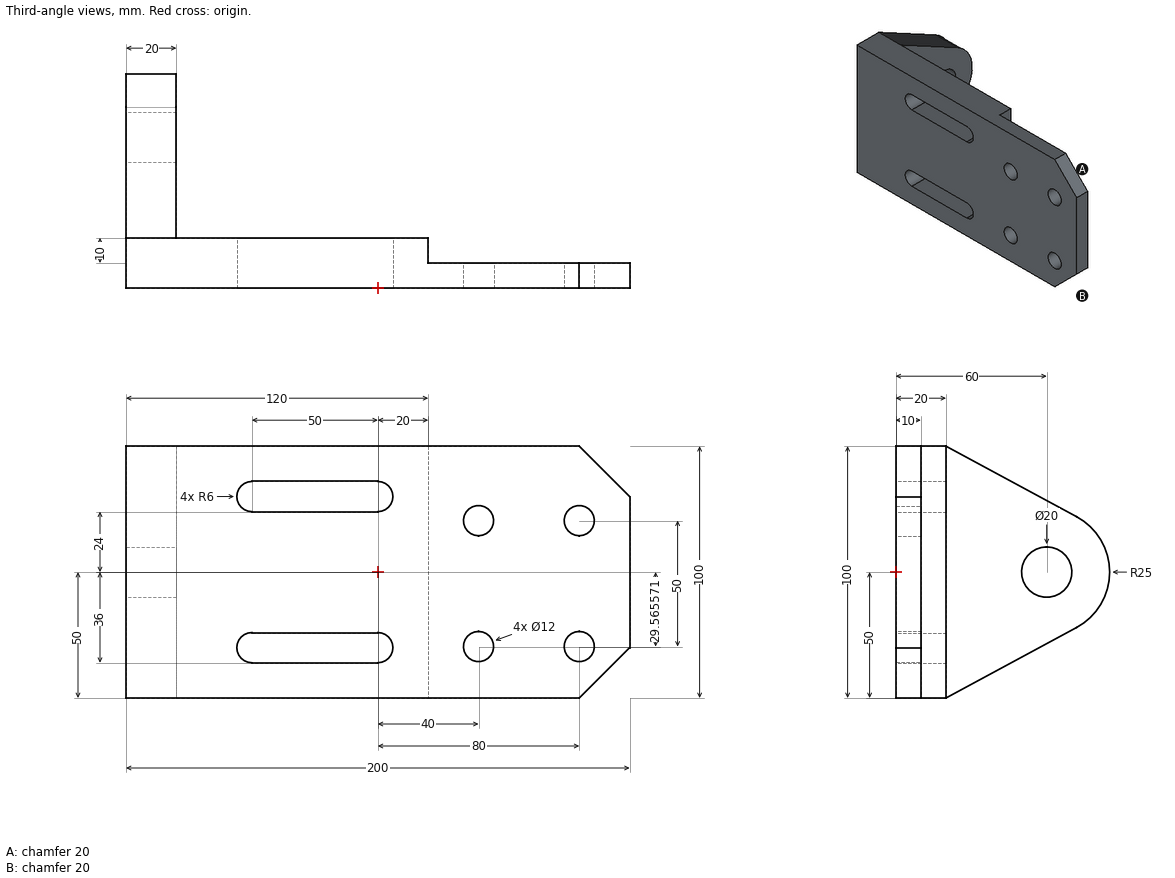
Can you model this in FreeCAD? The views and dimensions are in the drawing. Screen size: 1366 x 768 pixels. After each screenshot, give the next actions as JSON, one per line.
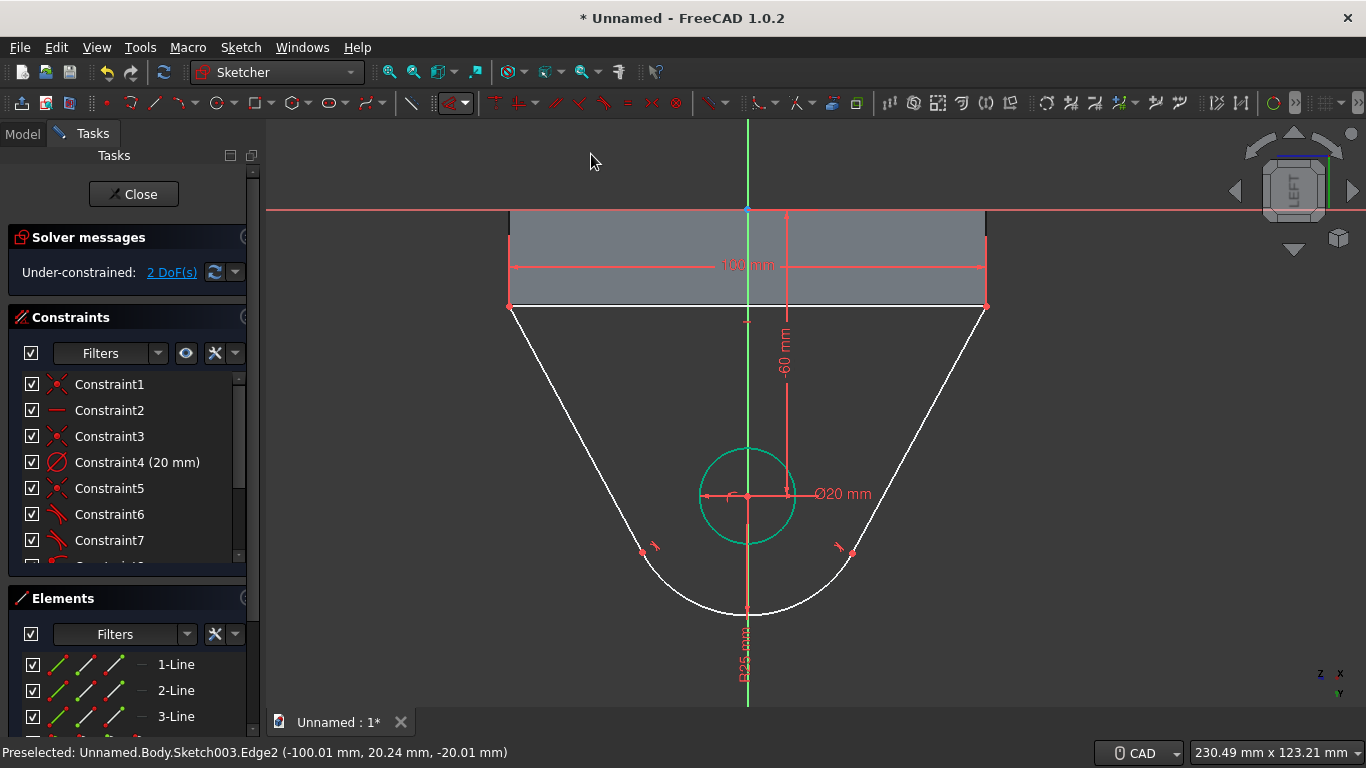
{"action": "left_click", "coordinate": [986, 306]}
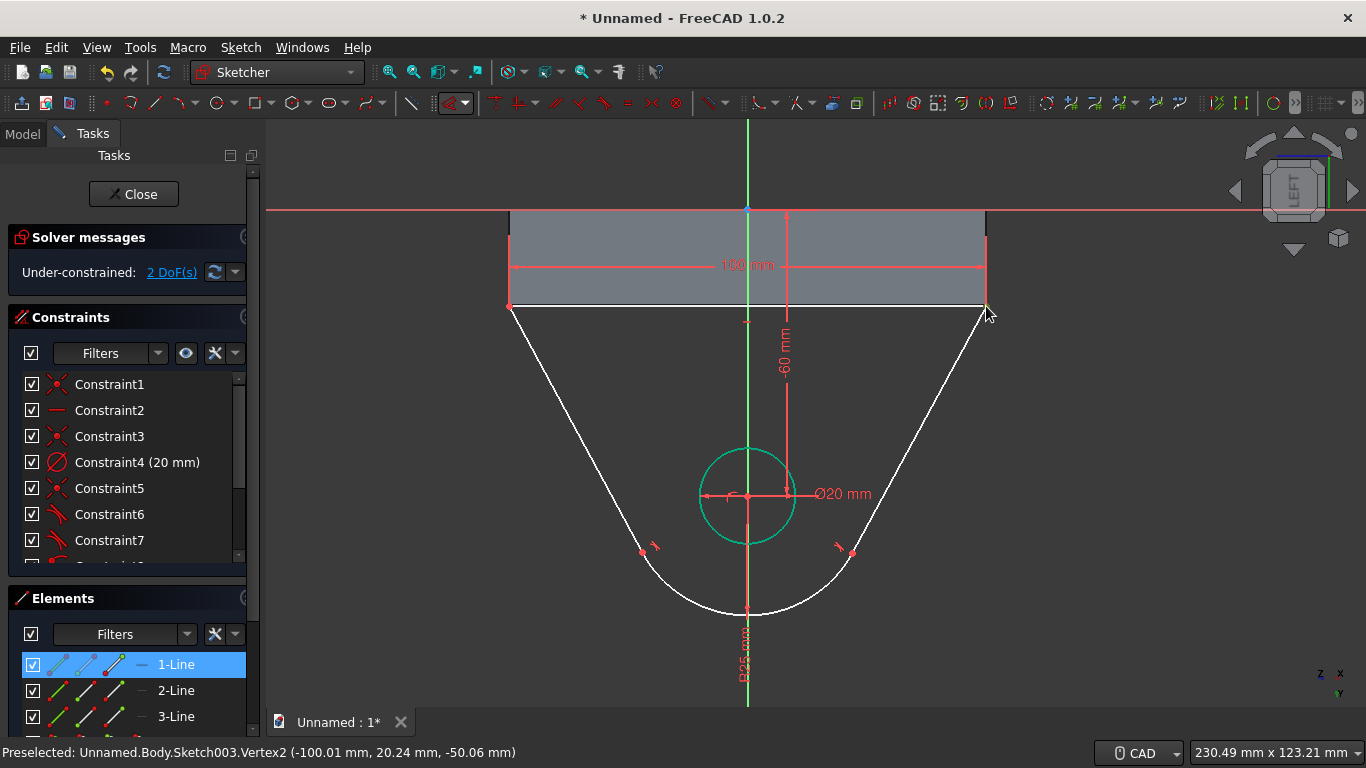
{"action": "key", "text": "l"}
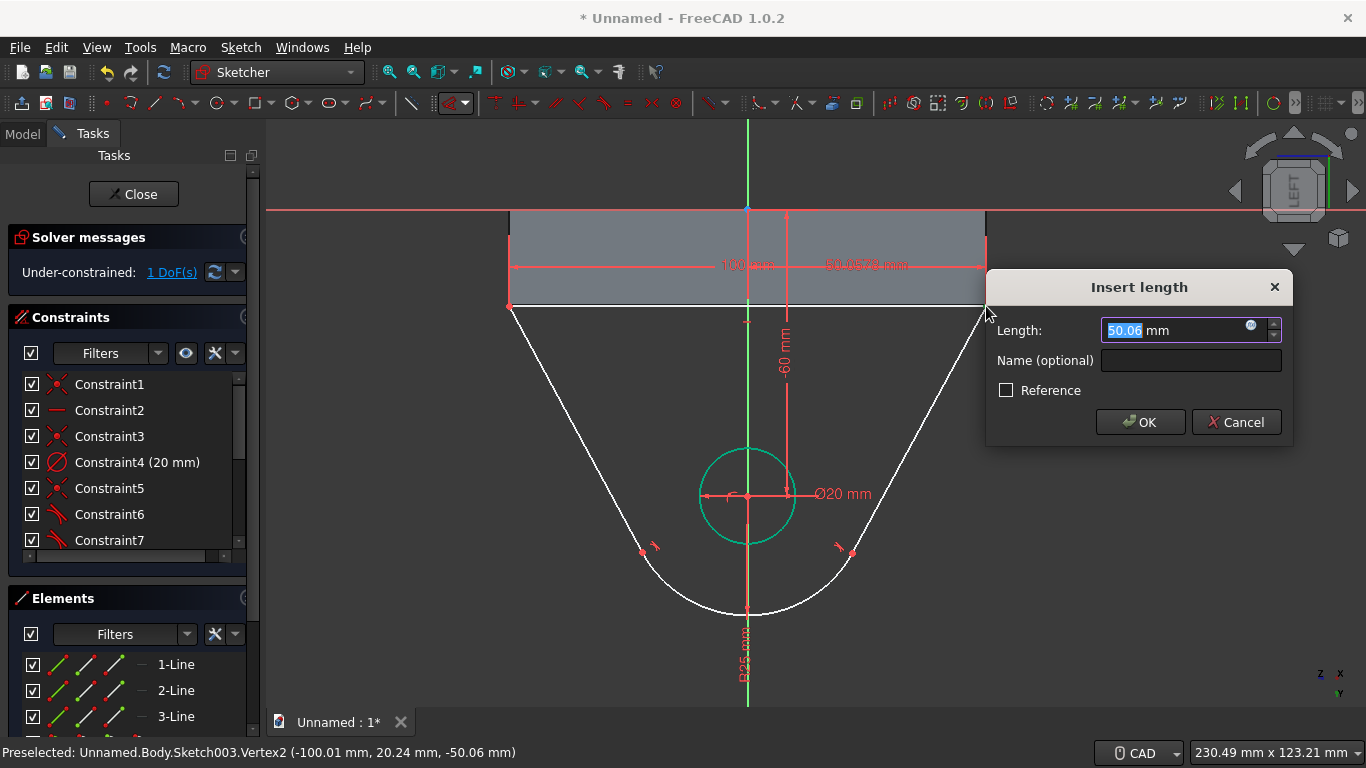
{"action": "type", "text": "50"}
{"action": "key", "text": "Return"}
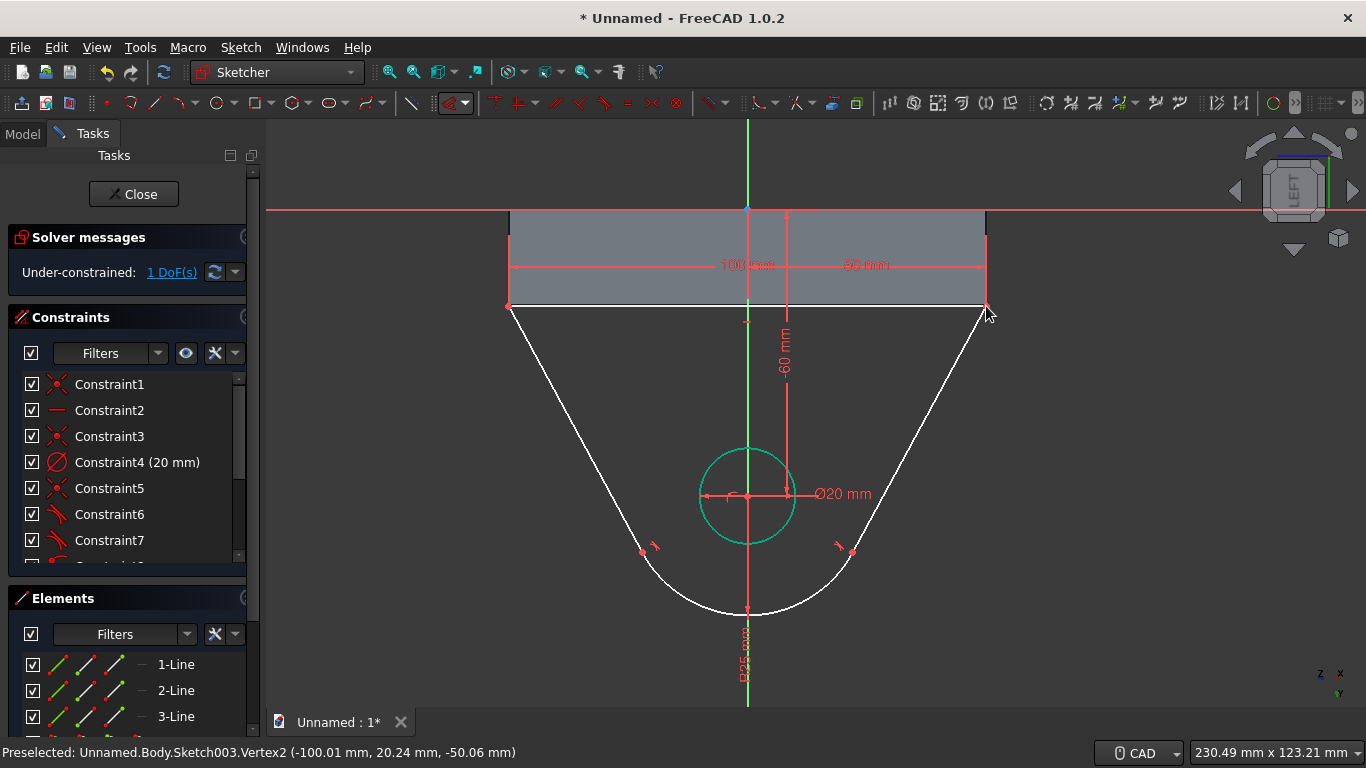
{"action": "left_click", "coordinate": [986, 306]}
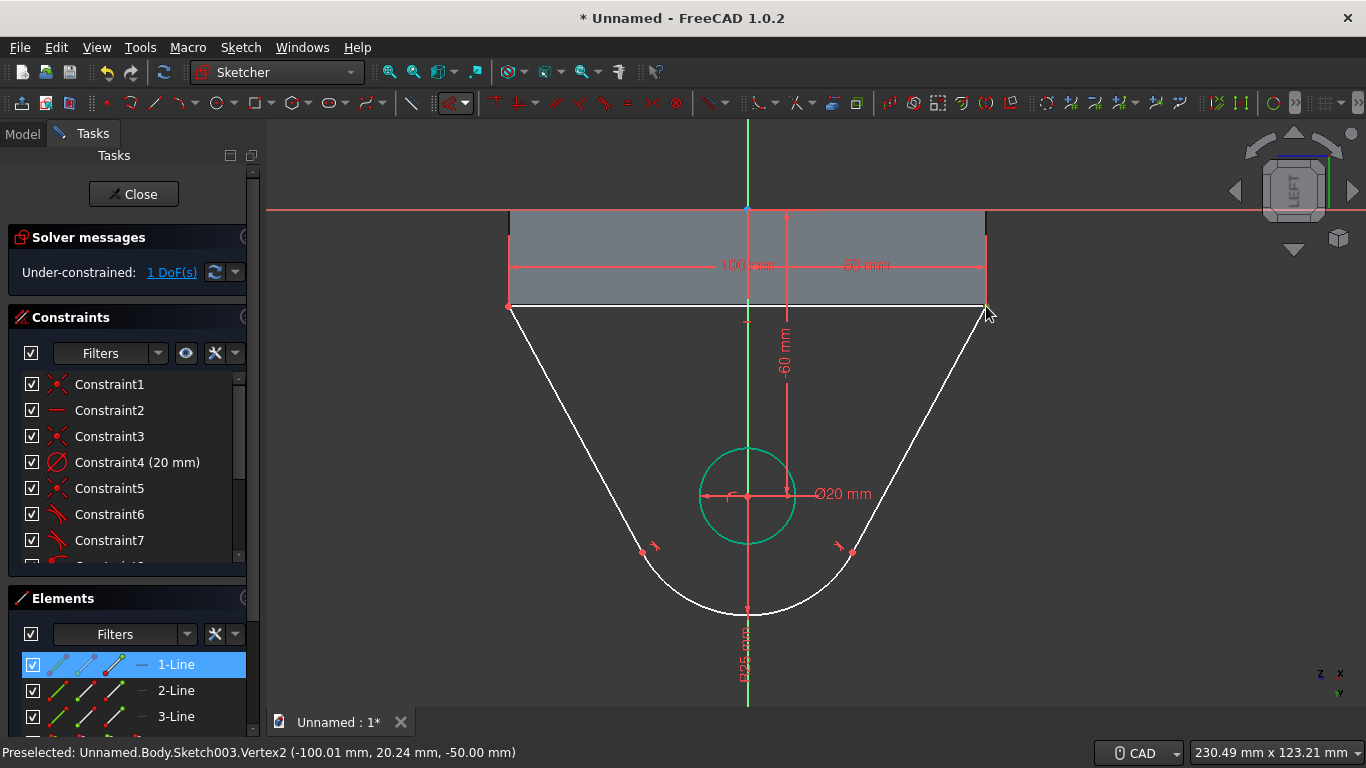
{"action": "left_click", "coordinate": [468, 104]}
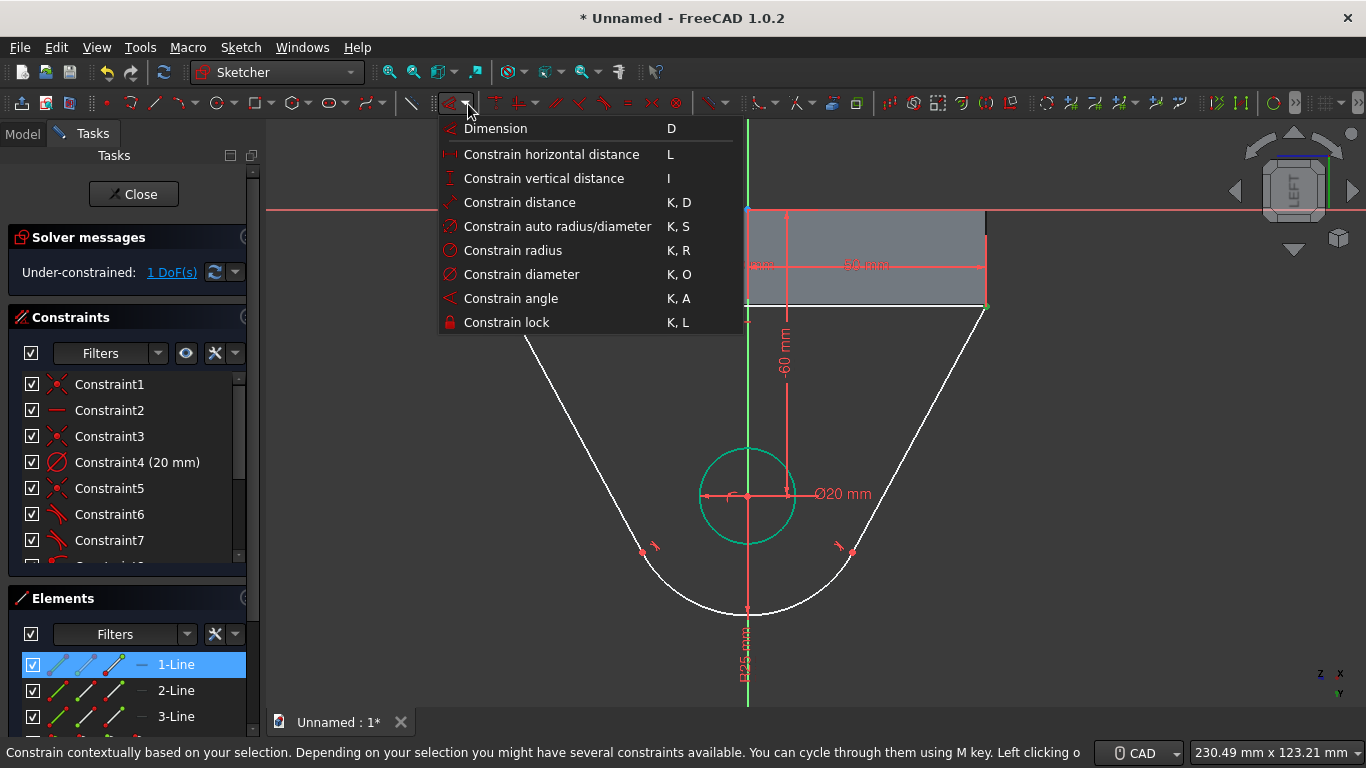
{"action": "left_click", "coordinate": [591, 178]}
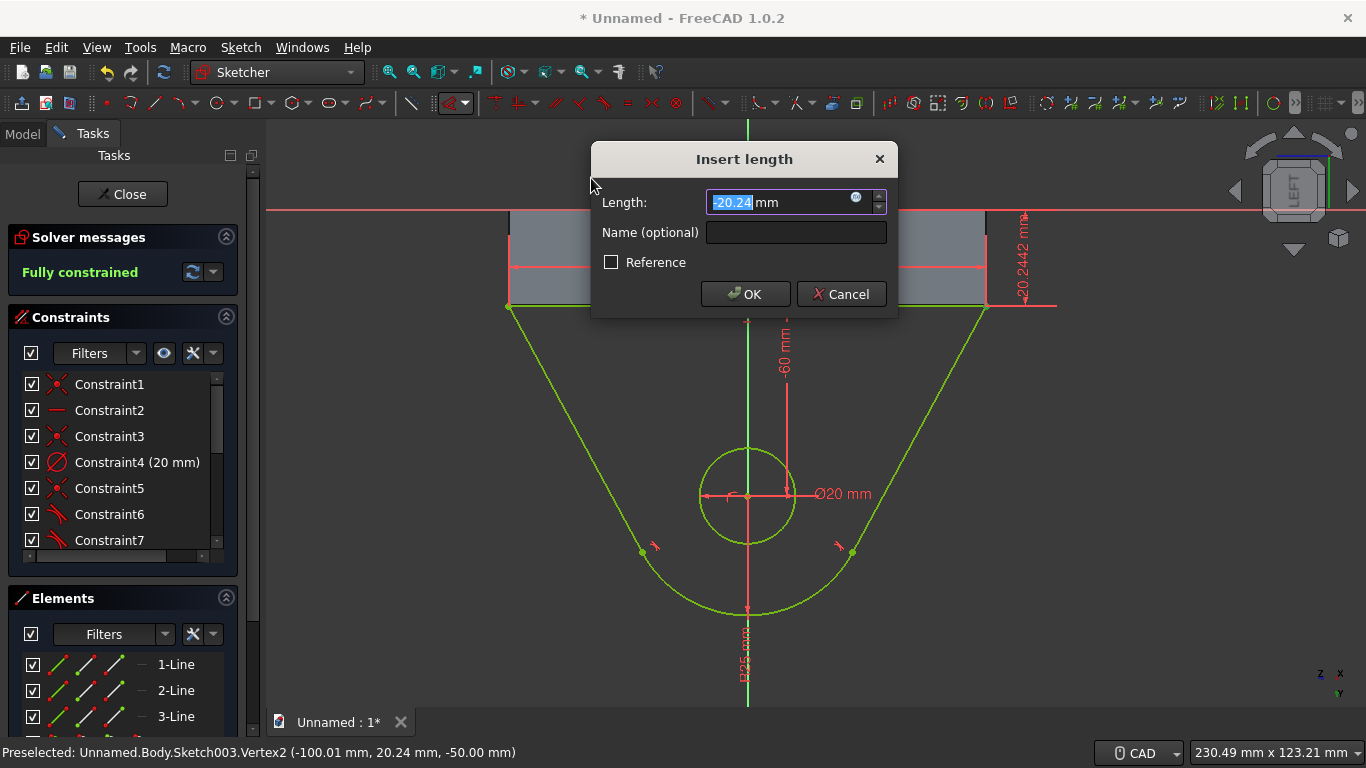
{"action": "type", "text": "-20"}
{"action": "key", "text": "Return"}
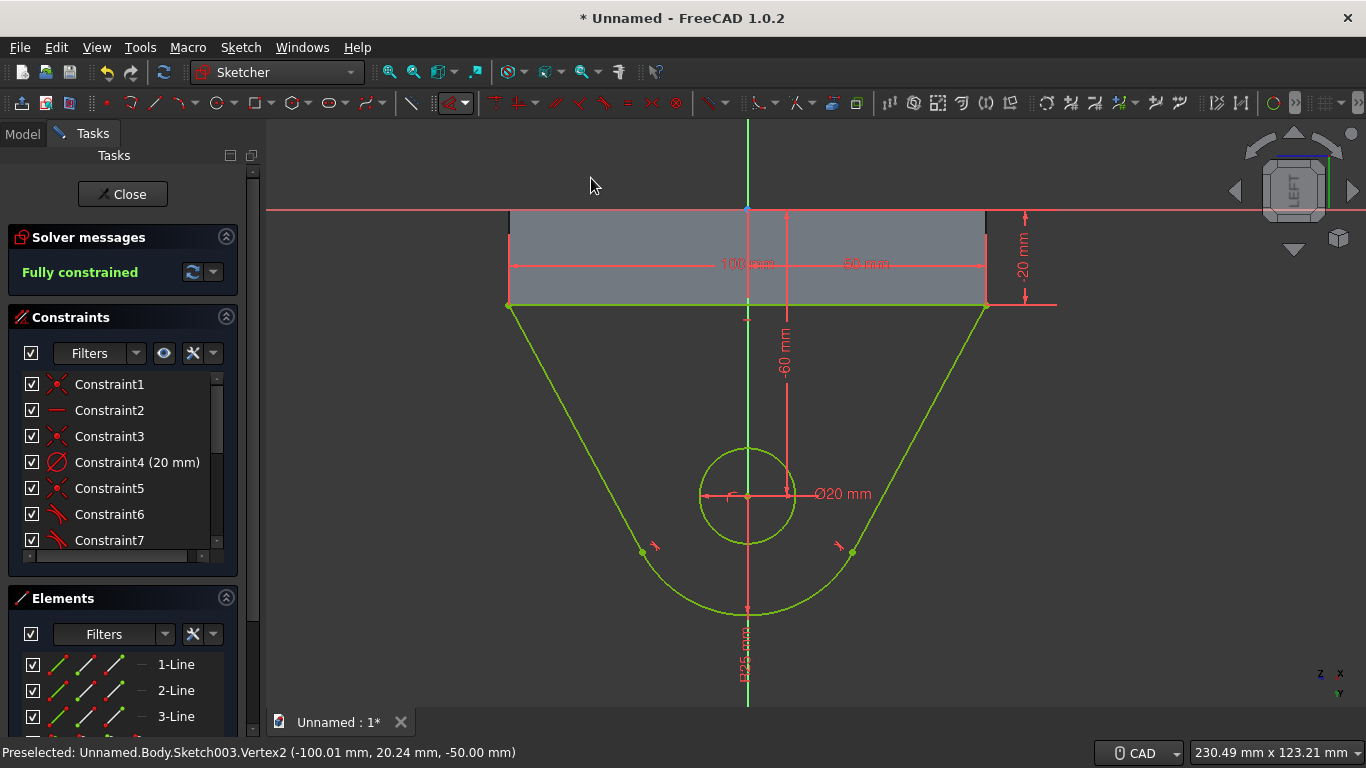
{"action": "left_click", "coordinate": [123, 194]}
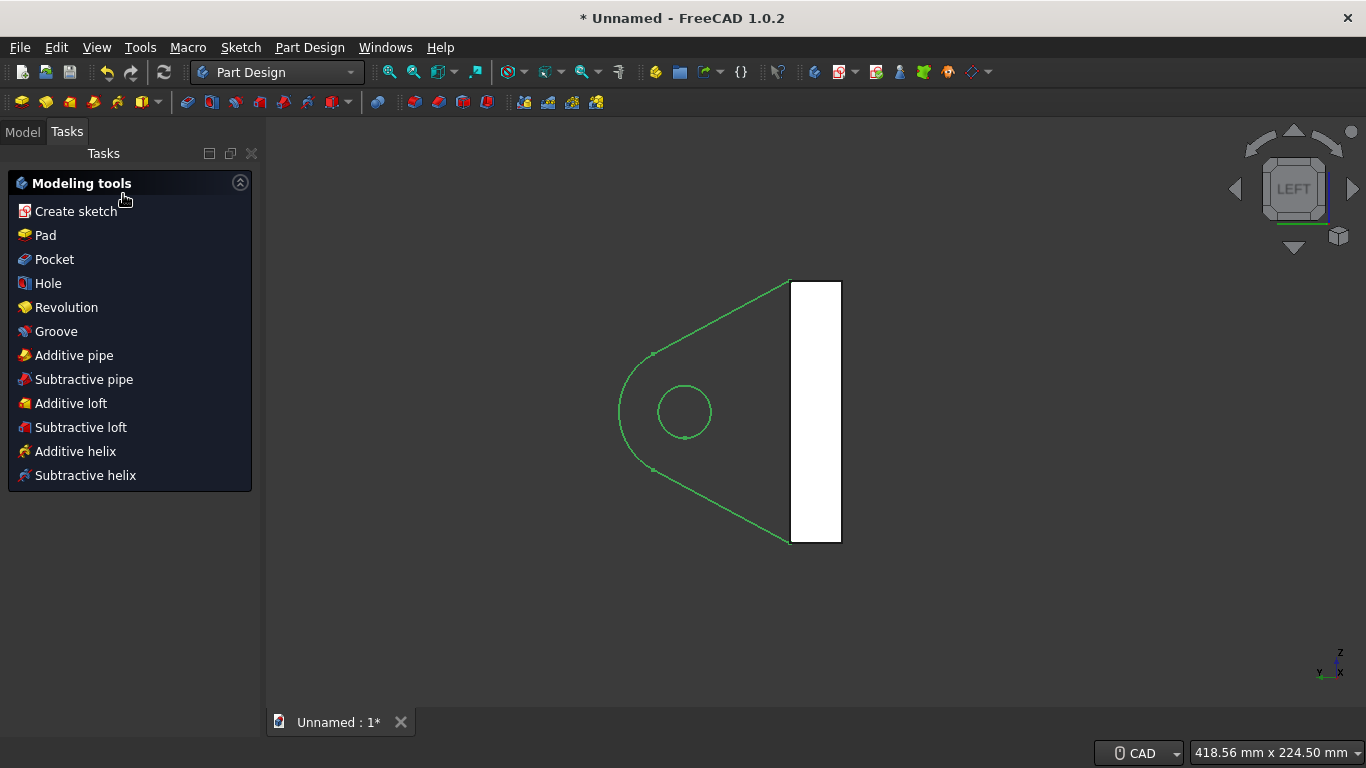
{"action": "left_click", "coordinate": [22, 102]}